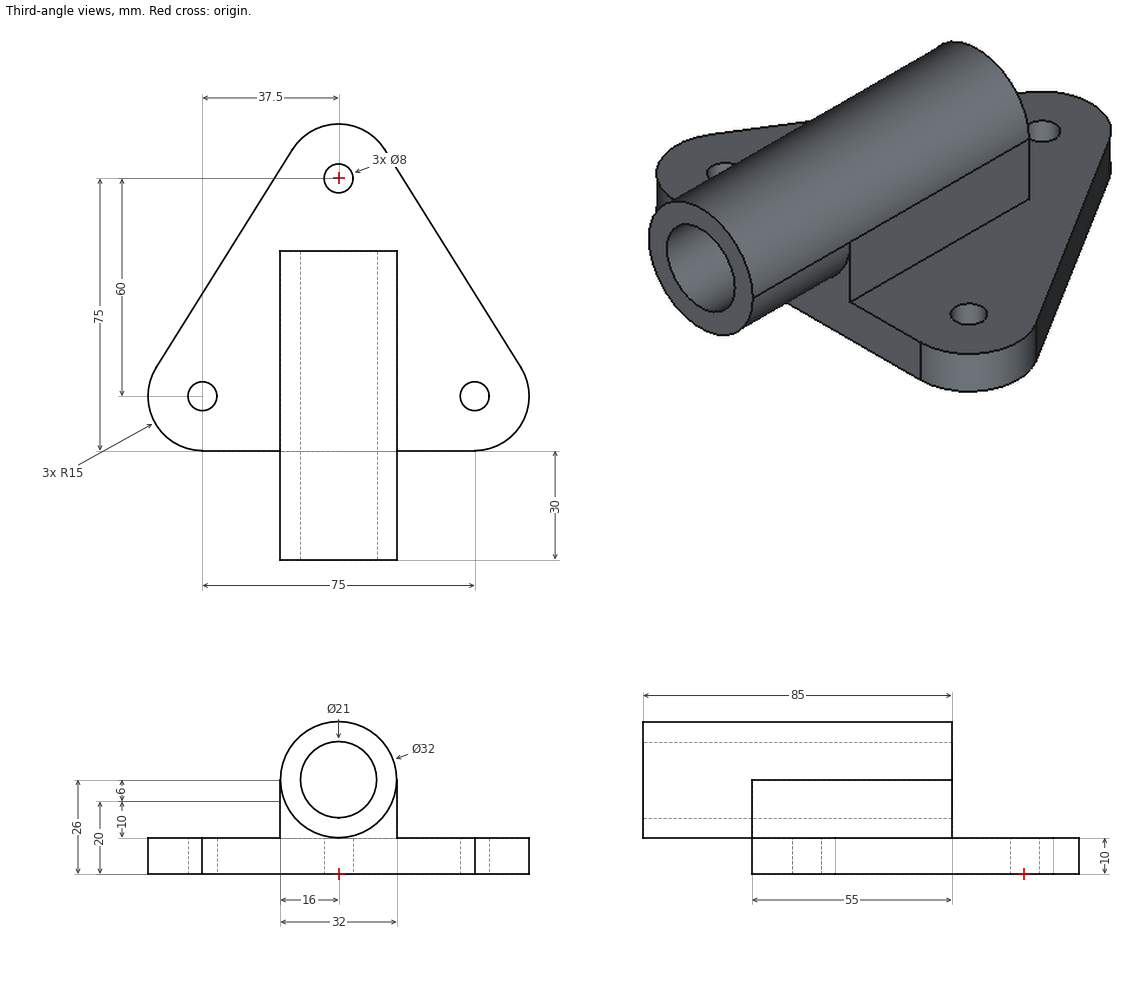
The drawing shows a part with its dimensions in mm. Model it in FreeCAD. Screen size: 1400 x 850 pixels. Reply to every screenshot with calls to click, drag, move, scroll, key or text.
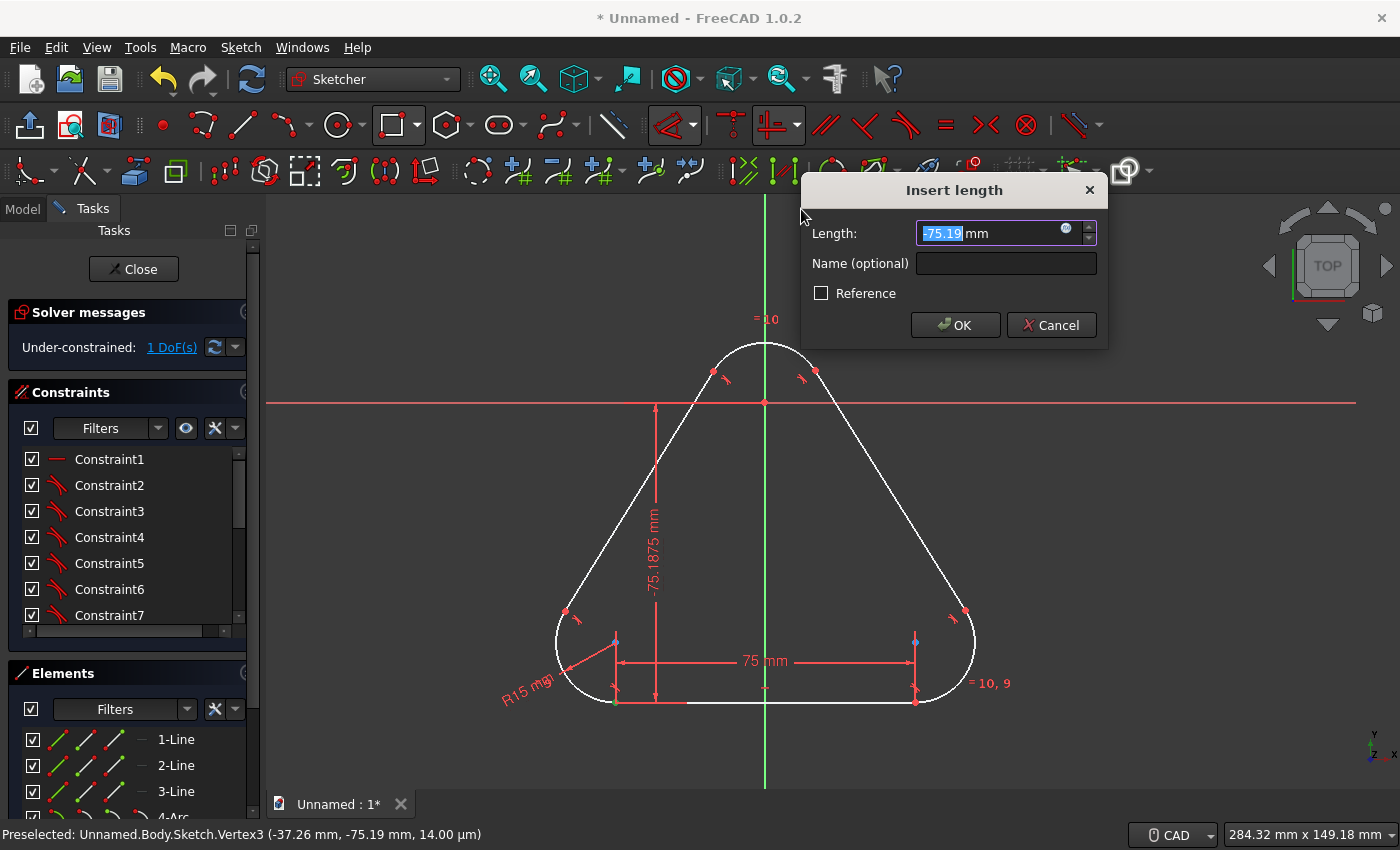
text(-75)
key(Return)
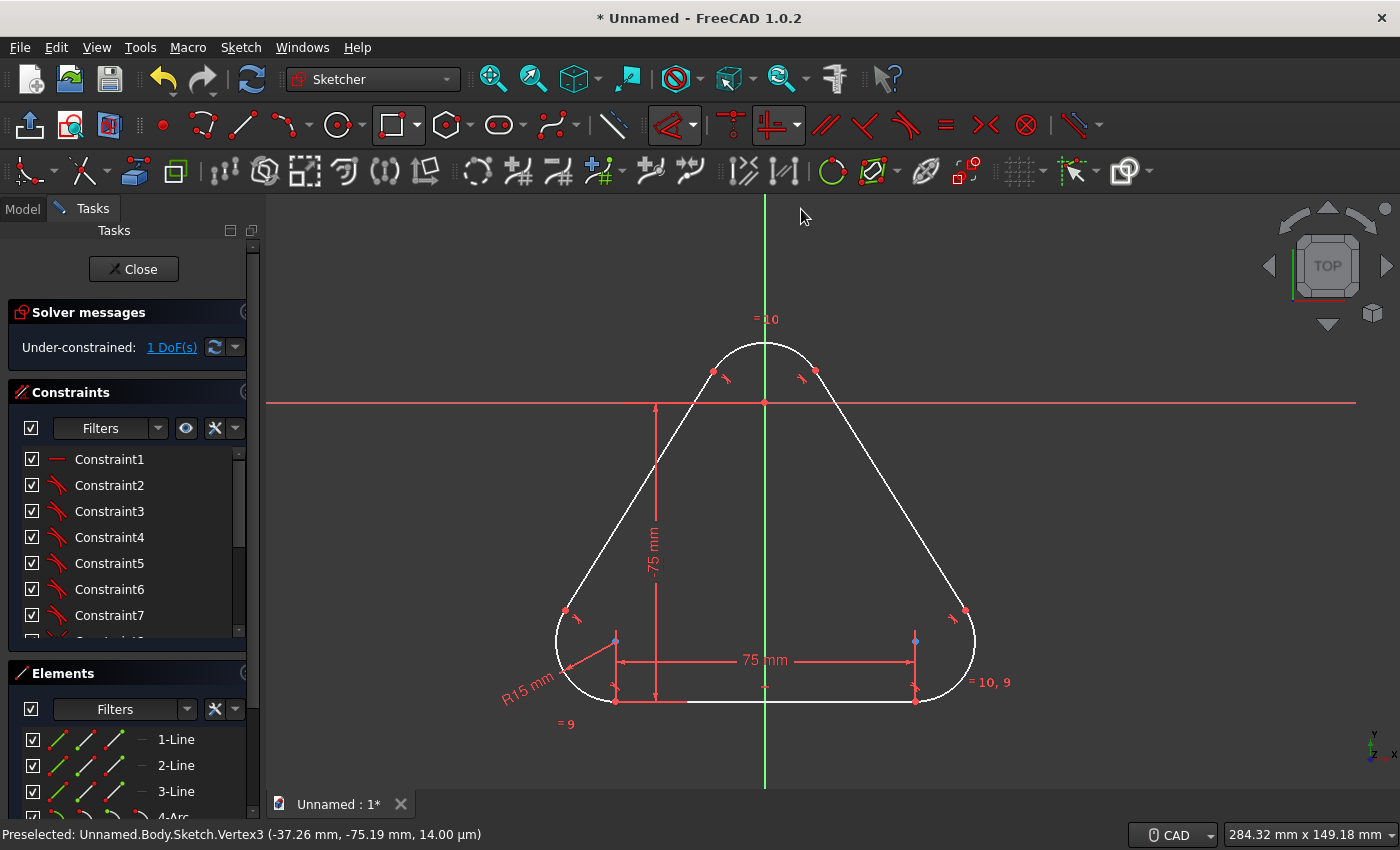
click(616, 702)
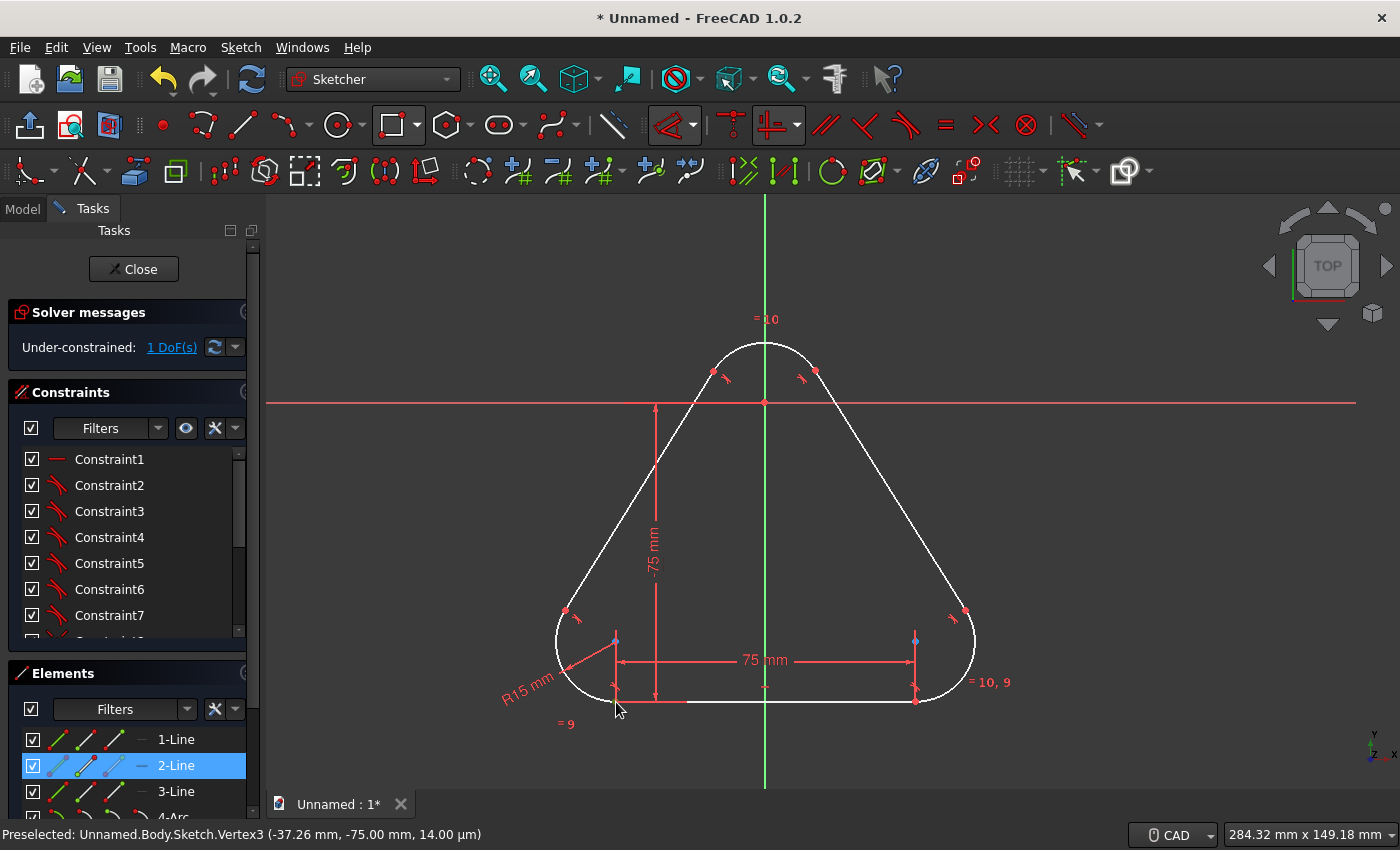
click(696, 126)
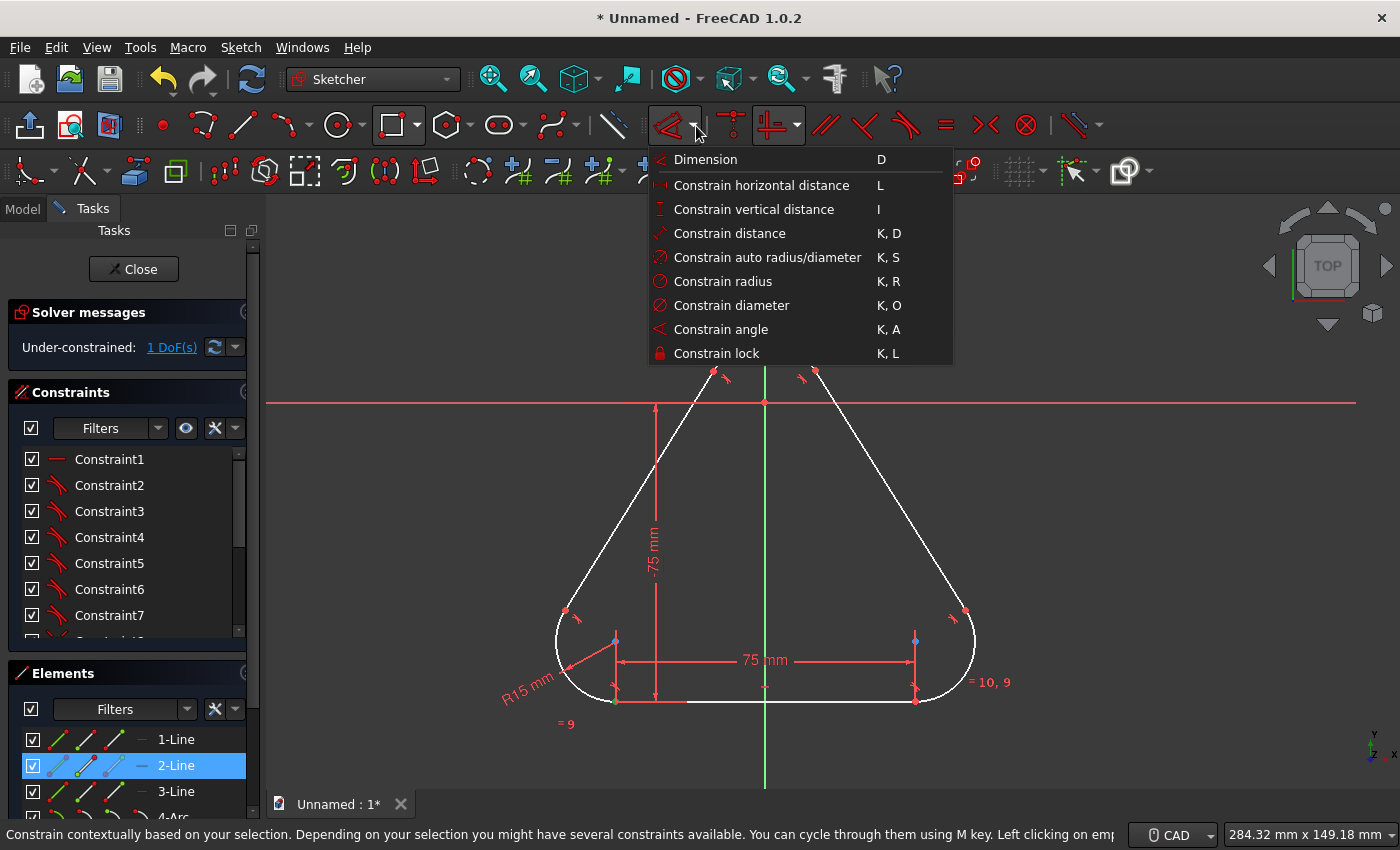
click(801, 185)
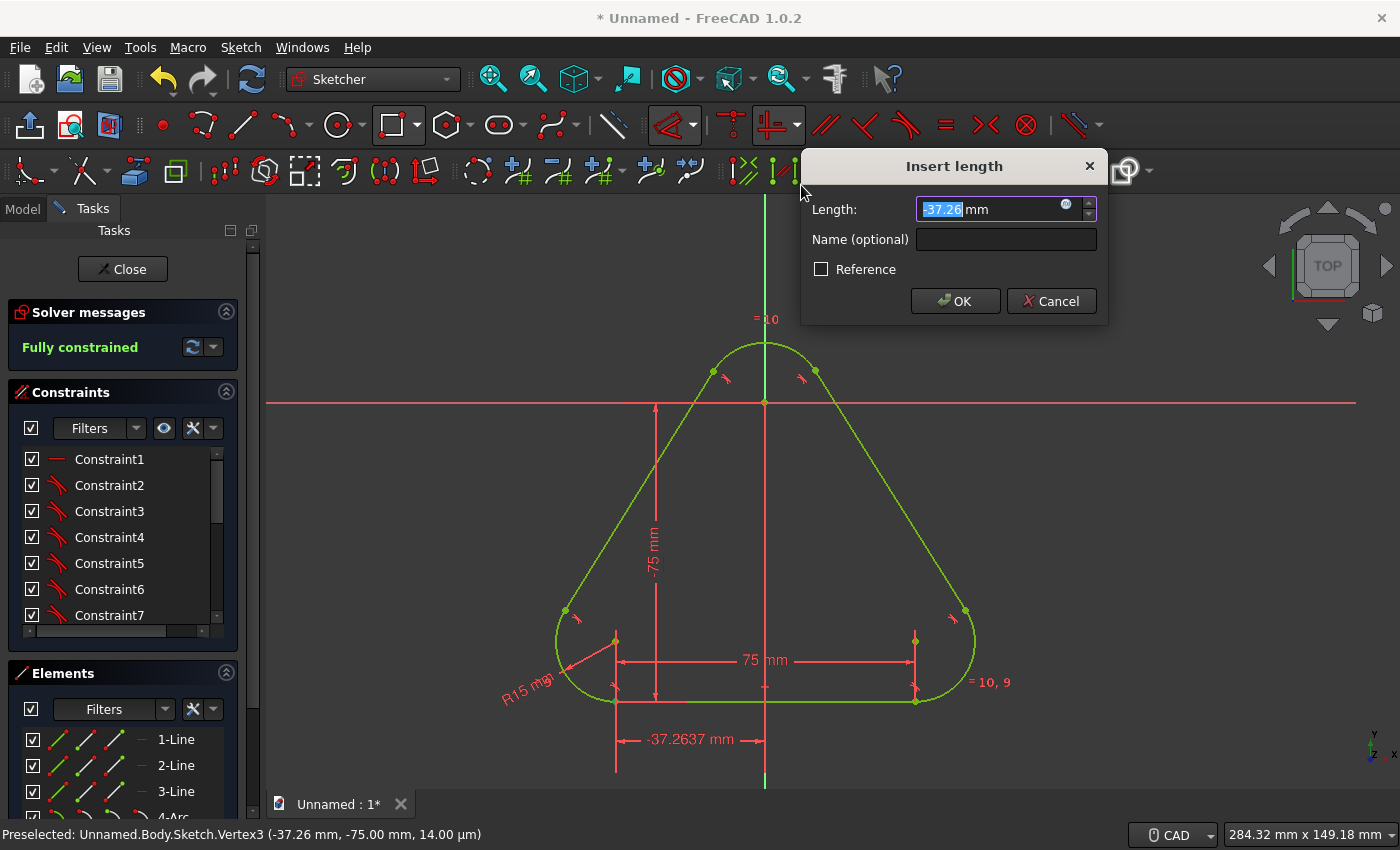
text(-37.5)
key(Return)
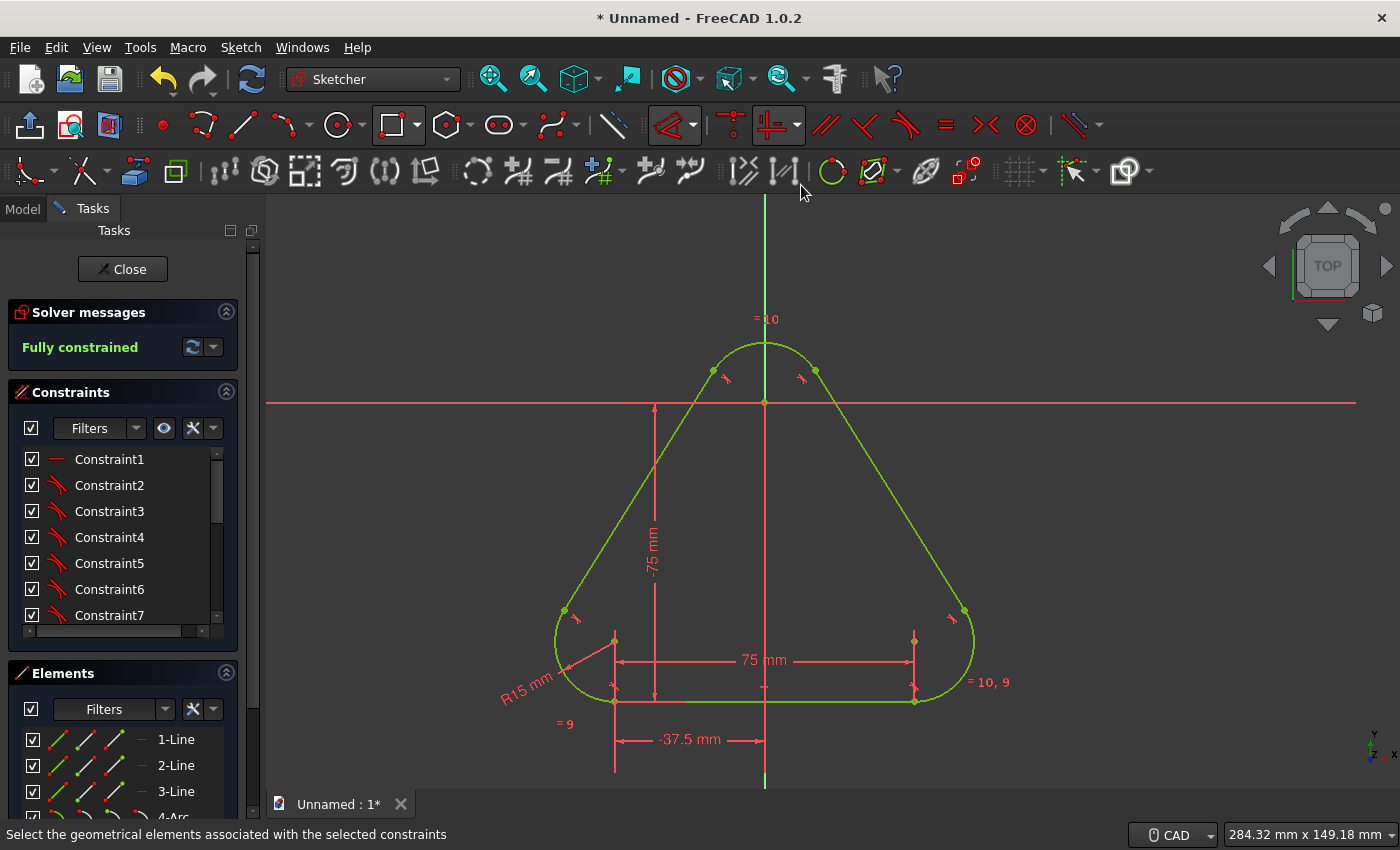
click(123, 269)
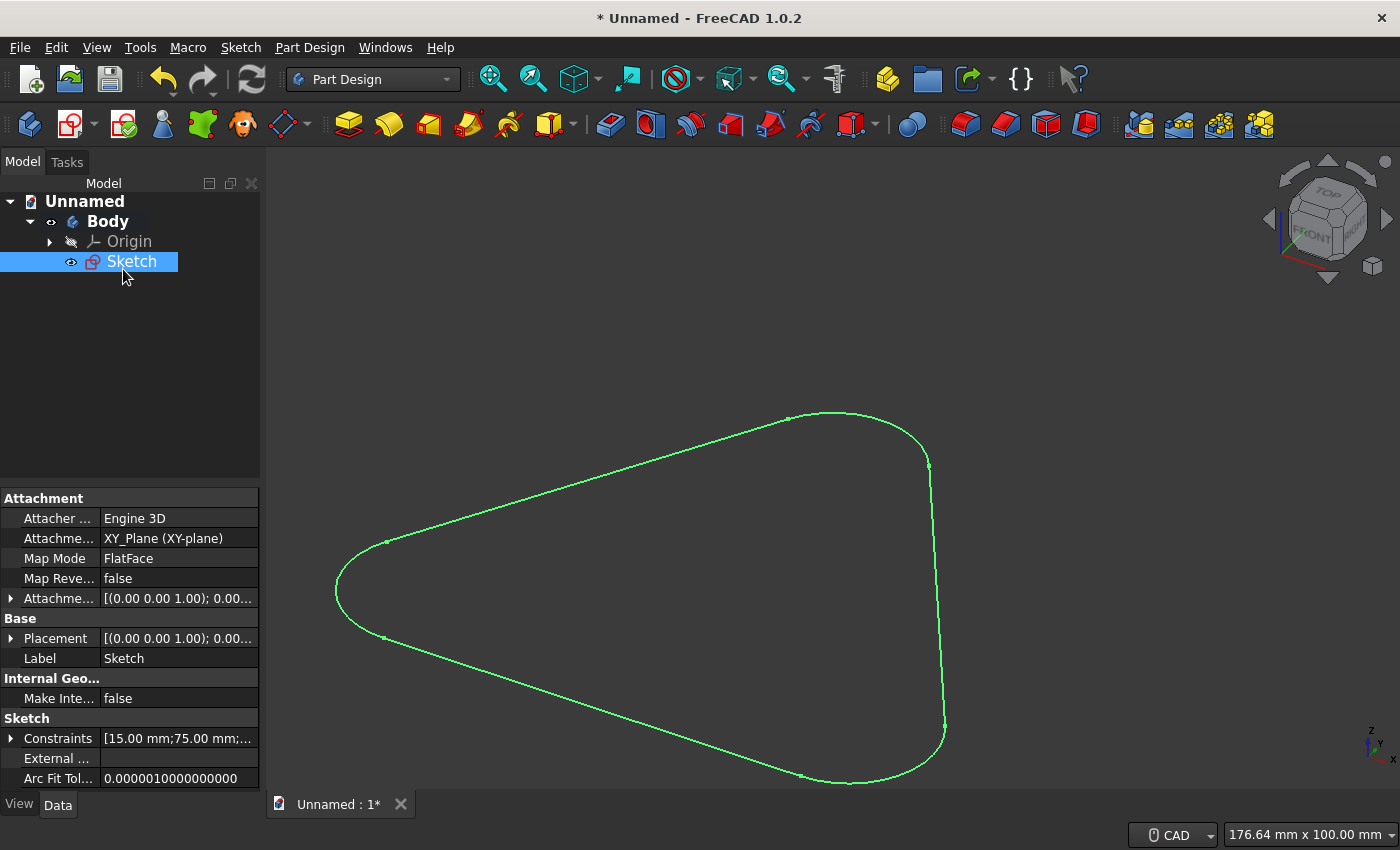
click(350, 124)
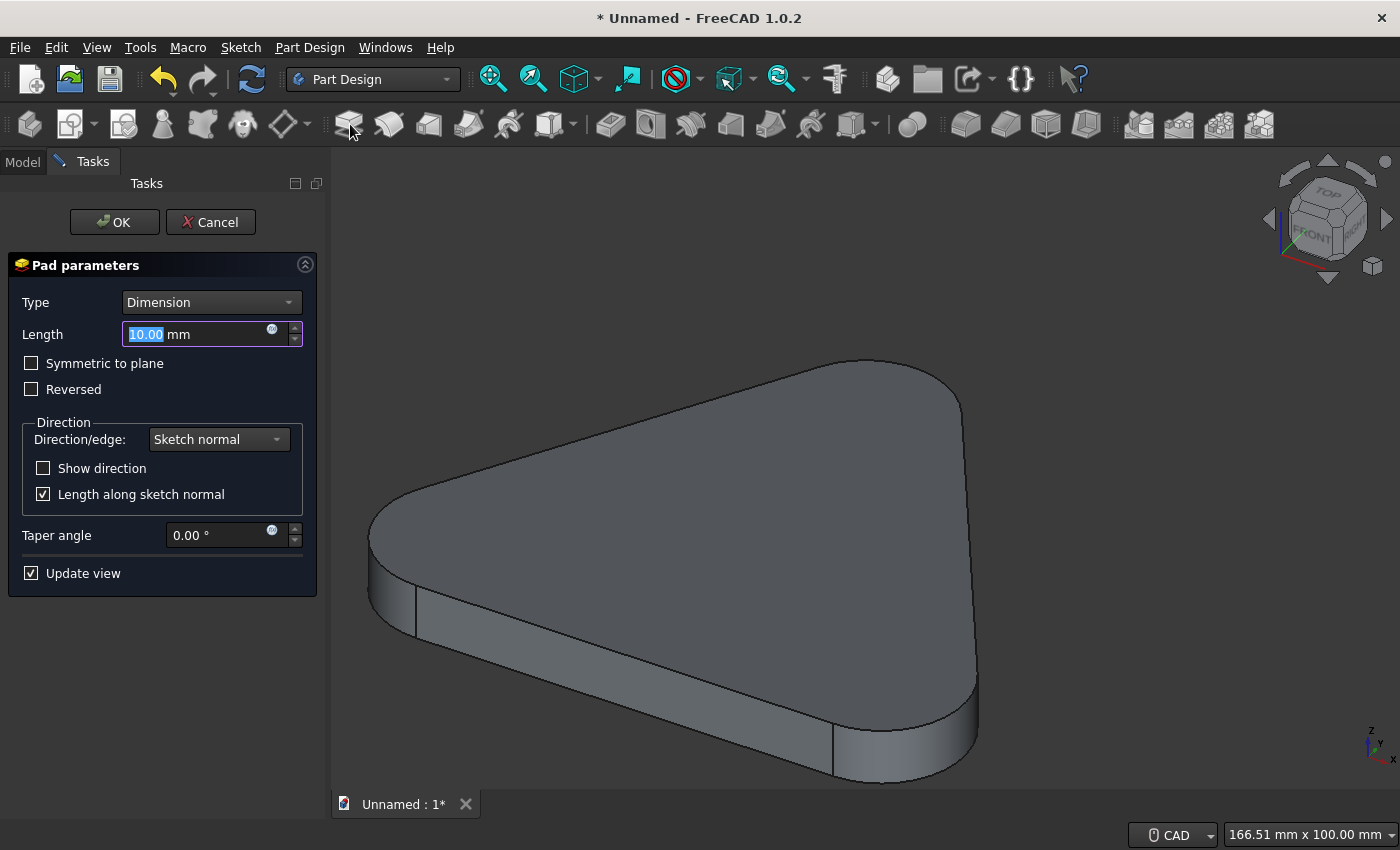
text(10)
key(Tab)